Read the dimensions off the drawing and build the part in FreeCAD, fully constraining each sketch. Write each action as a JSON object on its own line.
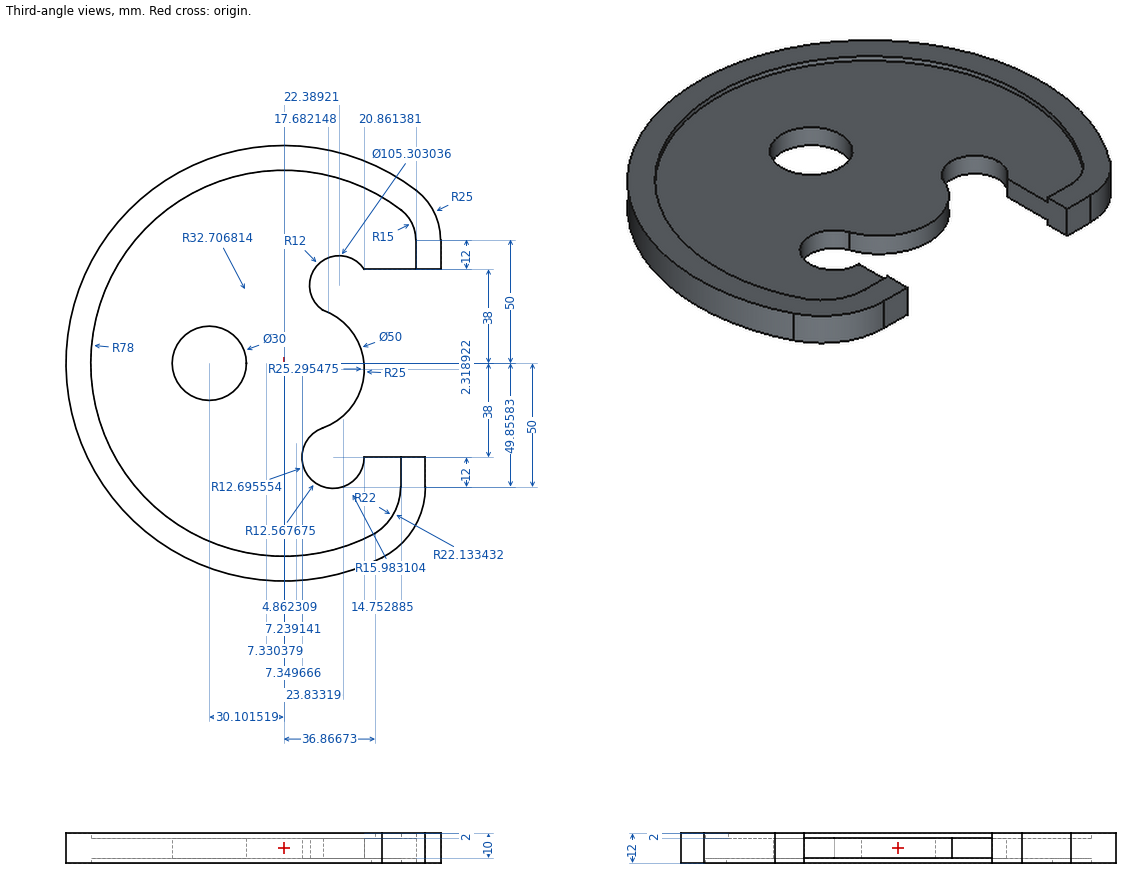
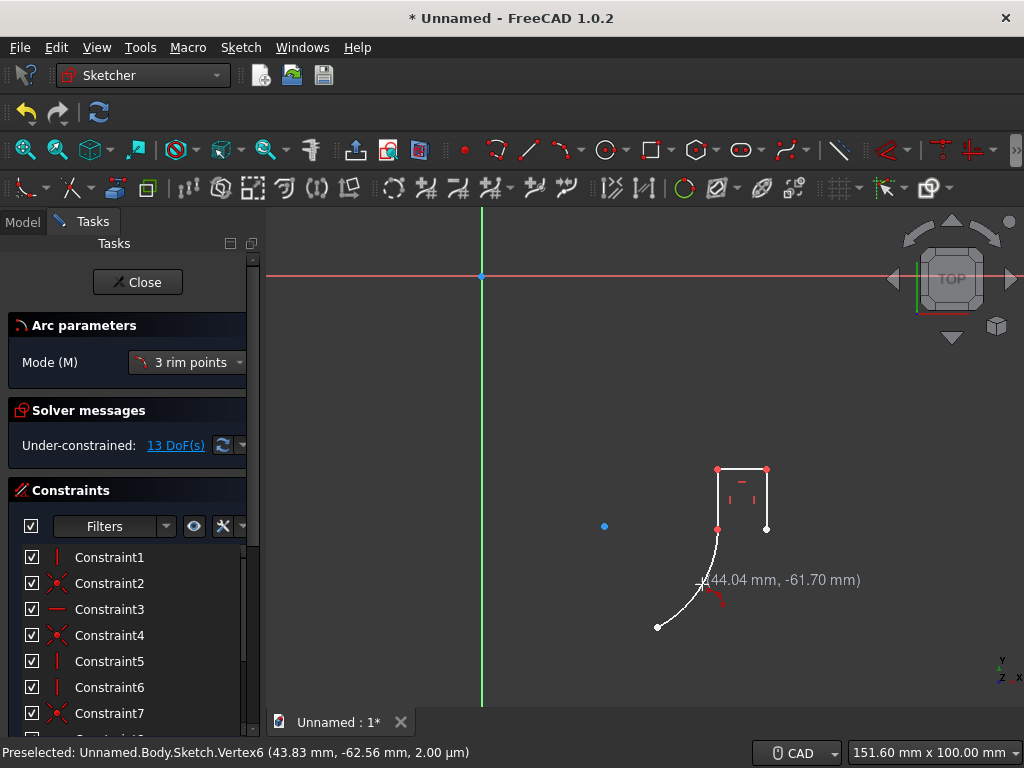
{"action": "left_click", "coordinate": [658, 627]}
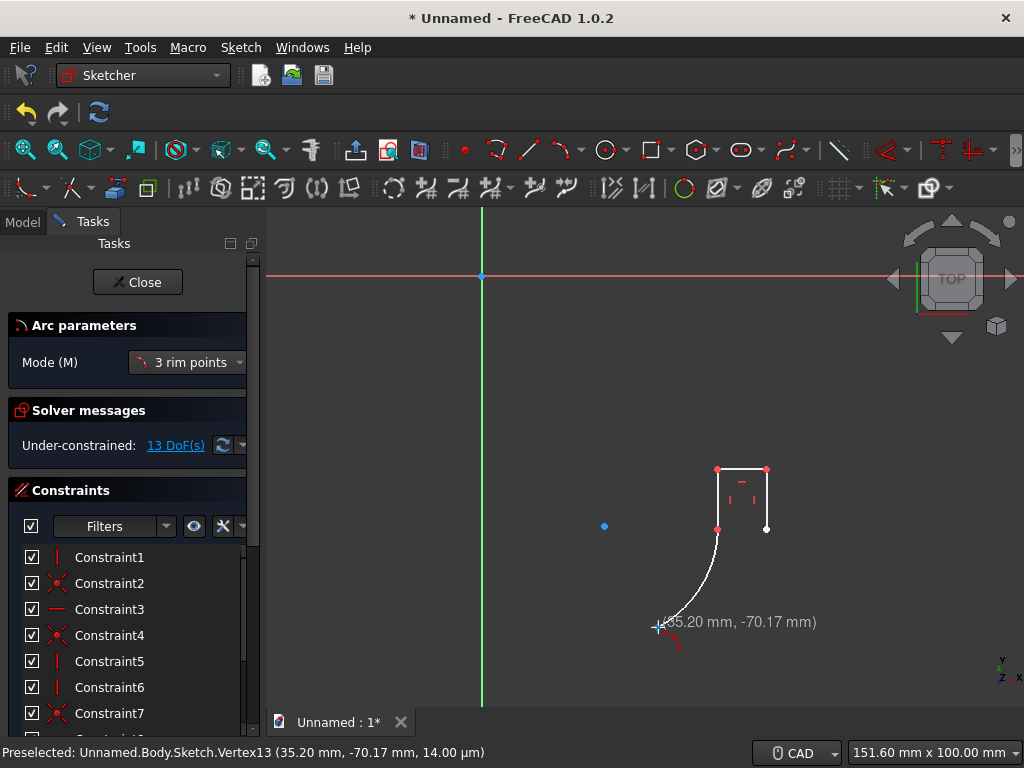
{"action": "scroll", "coordinate": [703, 586], "scroll_direction": "down", "scroll_amount": 4}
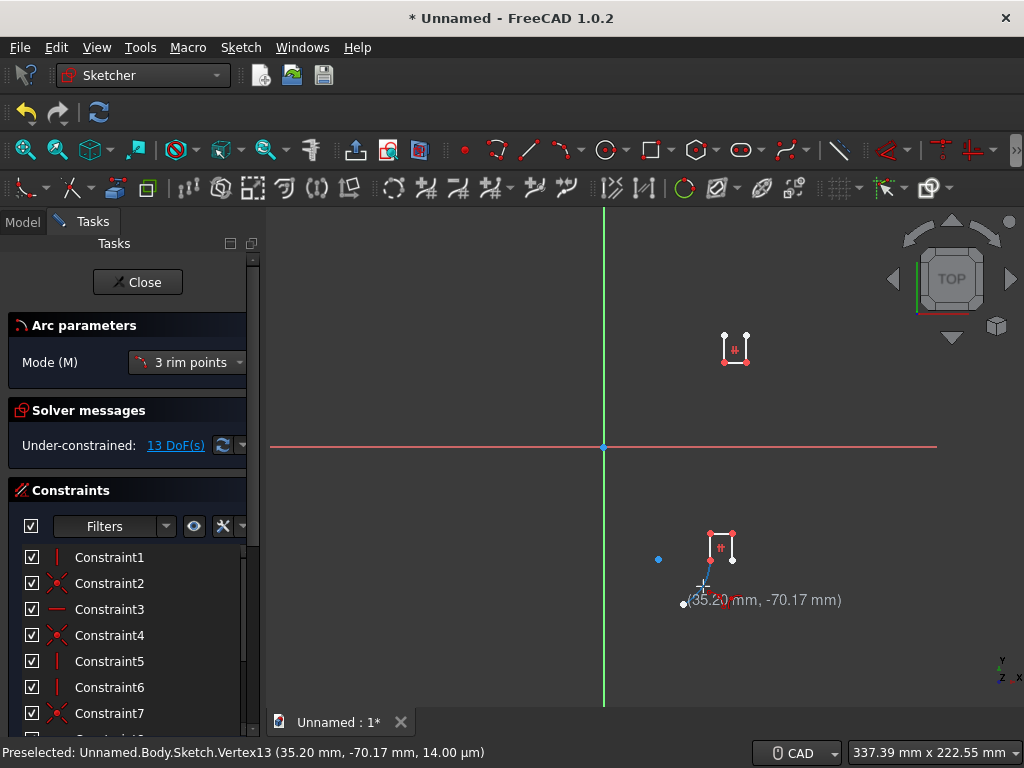
{"action": "left_click", "coordinate": [711, 308]}
{"action": "left_click", "coordinate": [429, 431]}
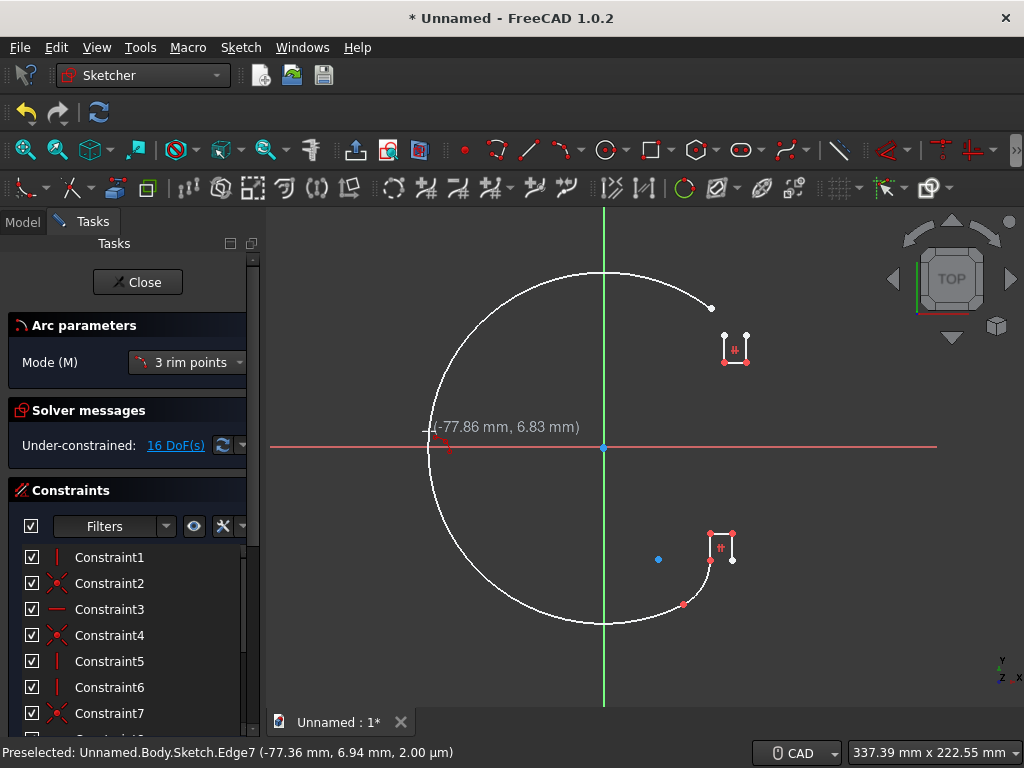
{"action": "left_click", "coordinate": [711, 309]}
{"action": "left_click", "coordinate": [724, 336]}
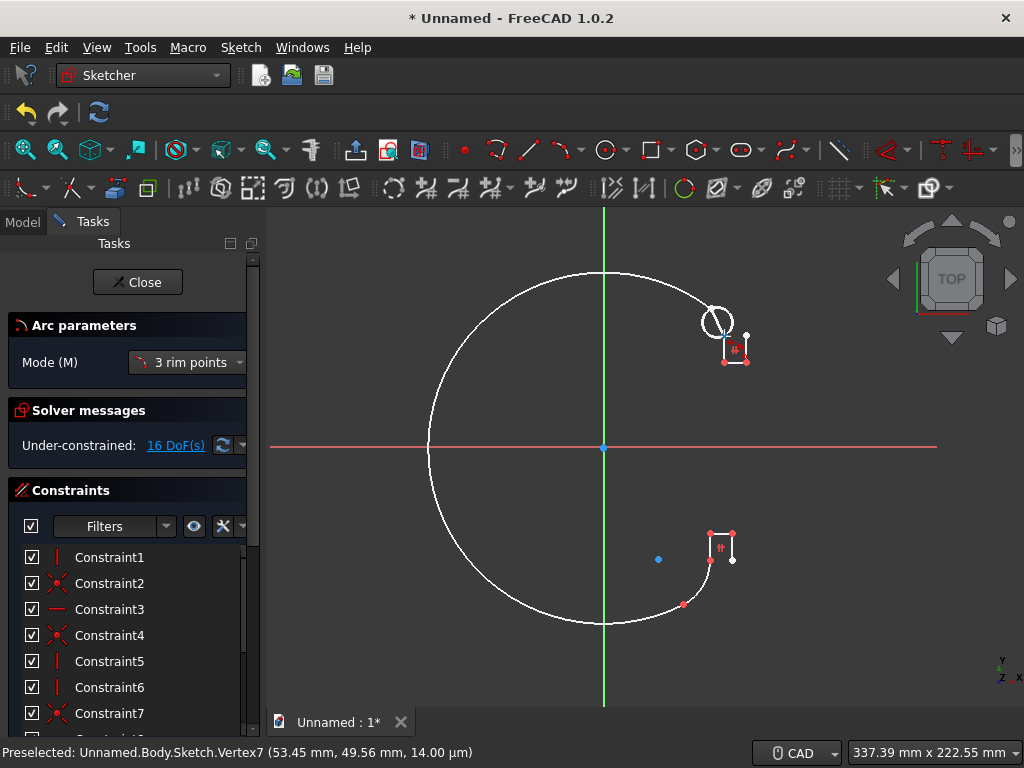
{"action": "scroll", "coordinate": [720, 320], "scroll_direction": "up", "scroll_amount": 8}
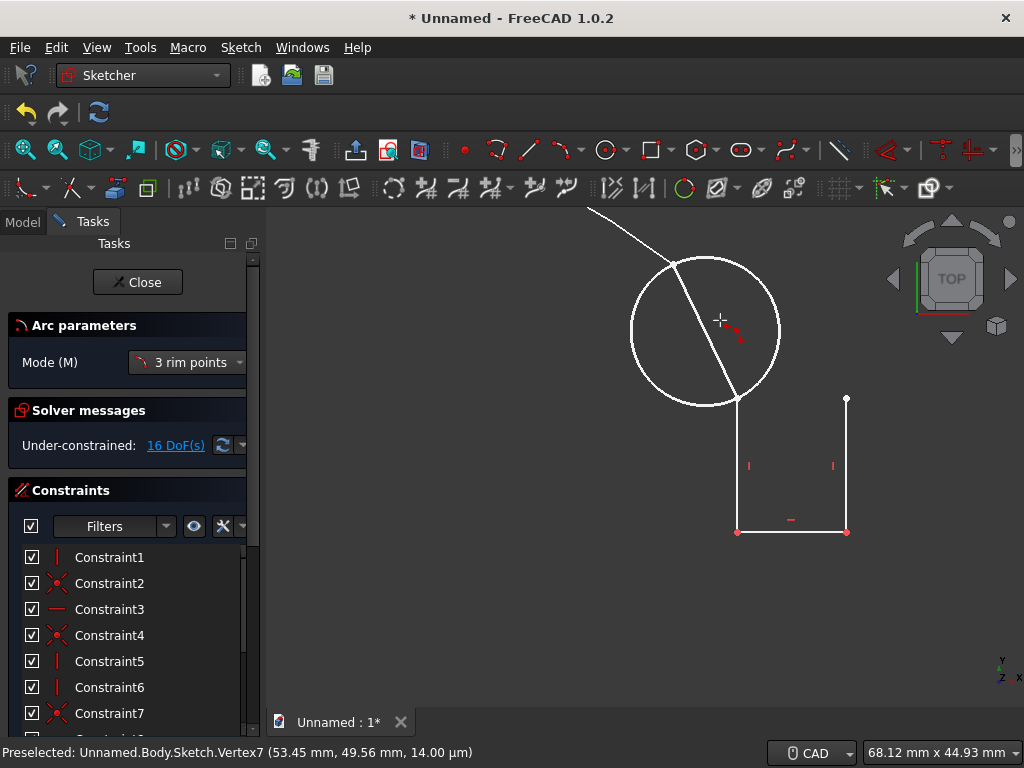
{"action": "left_click", "coordinate": [719, 320]}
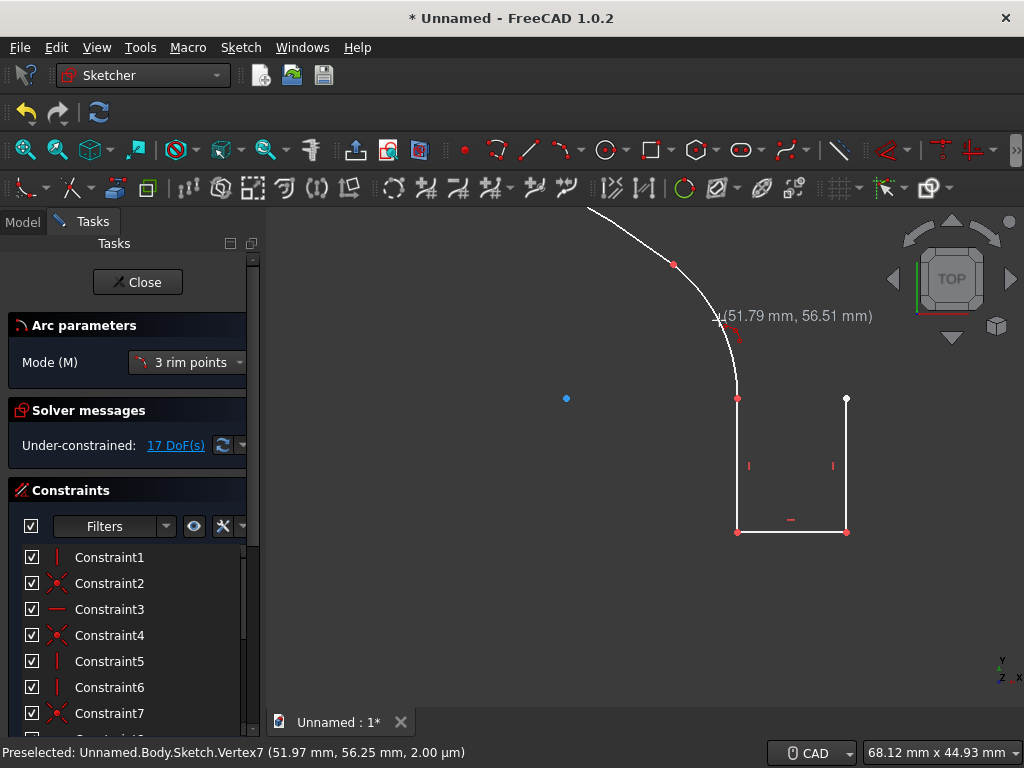
{"action": "scroll", "coordinate": [720, 320], "scroll_direction": "down", "scroll_amount": 8}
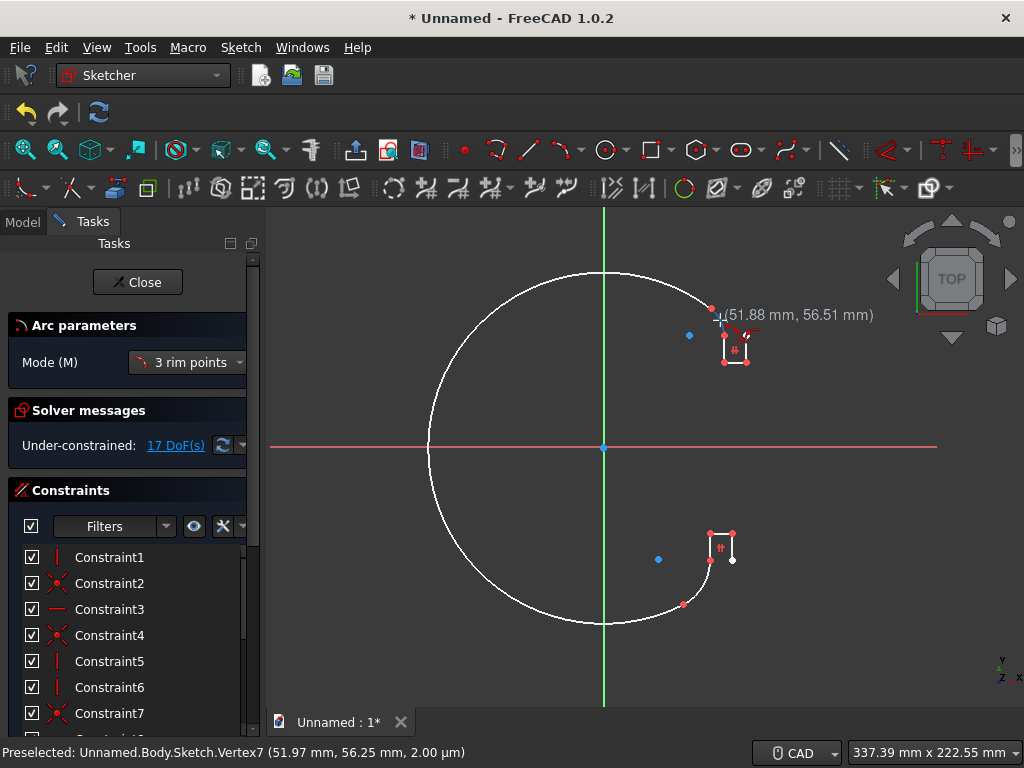
{"action": "left_click", "coordinate": [746, 336]}
{"action": "left_click", "coordinate": [724, 290]}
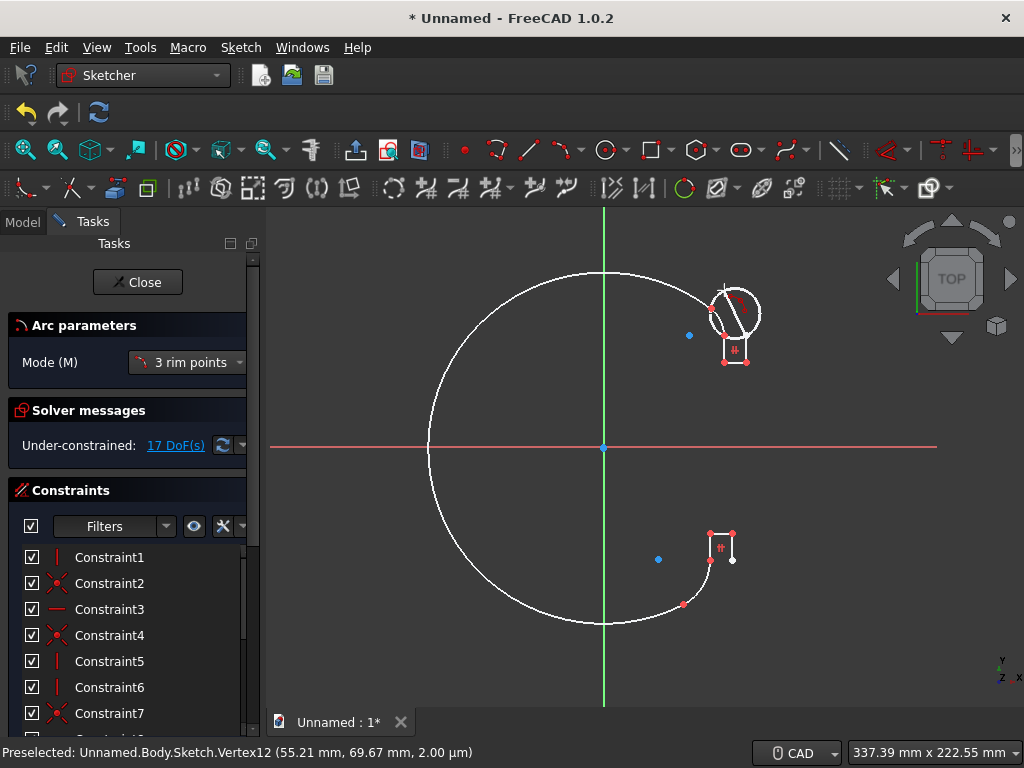
{"action": "scroll", "coordinate": [740, 310], "scroll_direction": "up", "scroll_amount": 6}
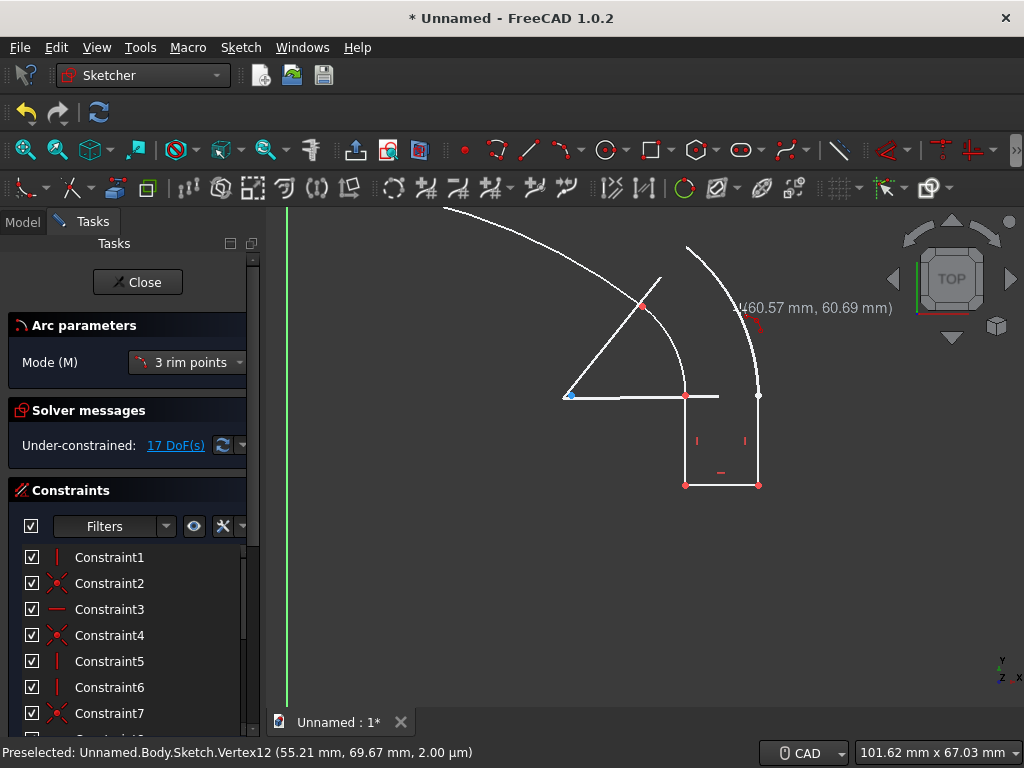
{"action": "left_click", "coordinate": [740, 310]}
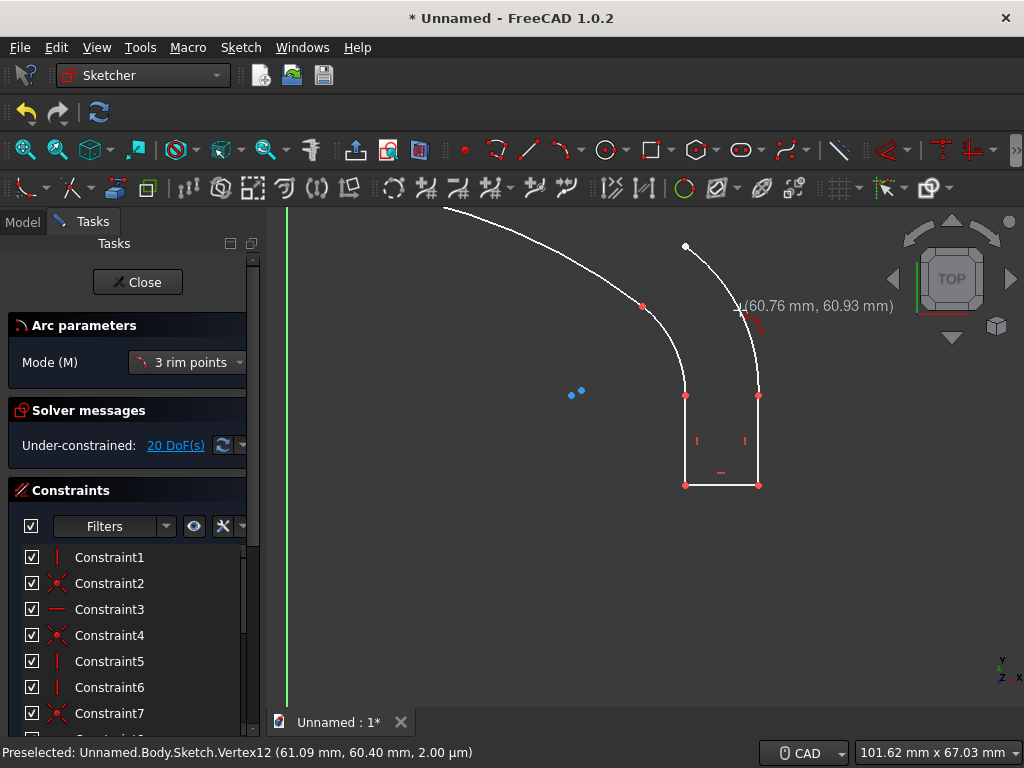
{"action": "left_click", "coordinate": [685, 246]}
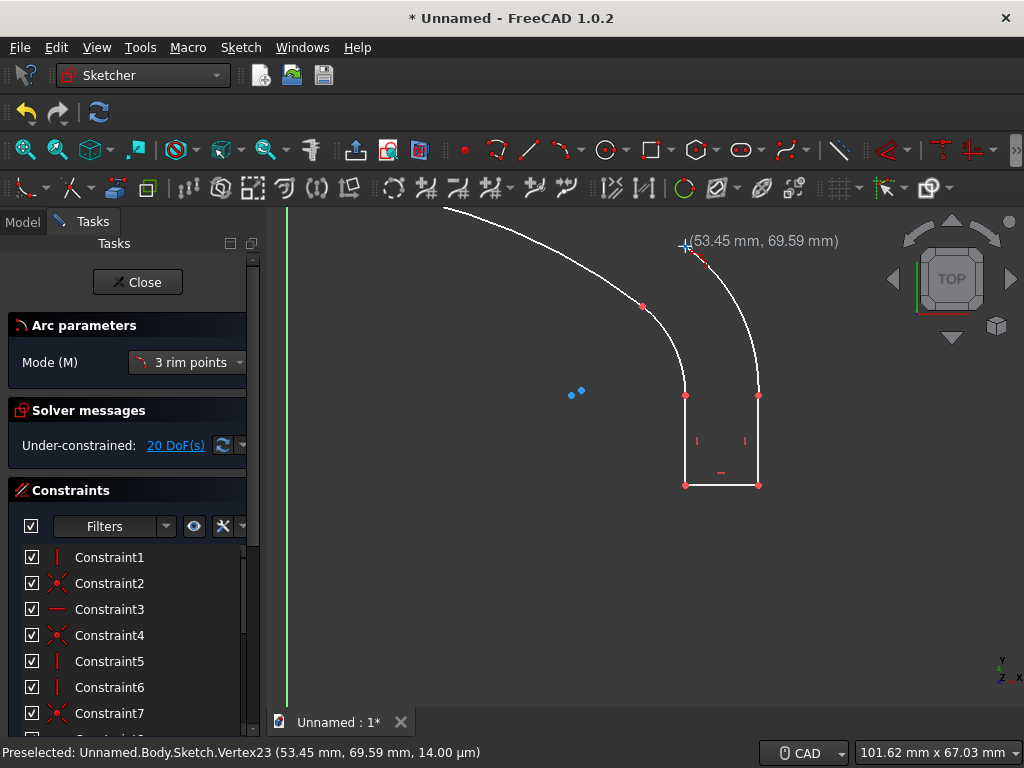
{"action": "scroll", "coordinate": [740, 310], "scroll_direction": "down", "scroll_amount": 6}